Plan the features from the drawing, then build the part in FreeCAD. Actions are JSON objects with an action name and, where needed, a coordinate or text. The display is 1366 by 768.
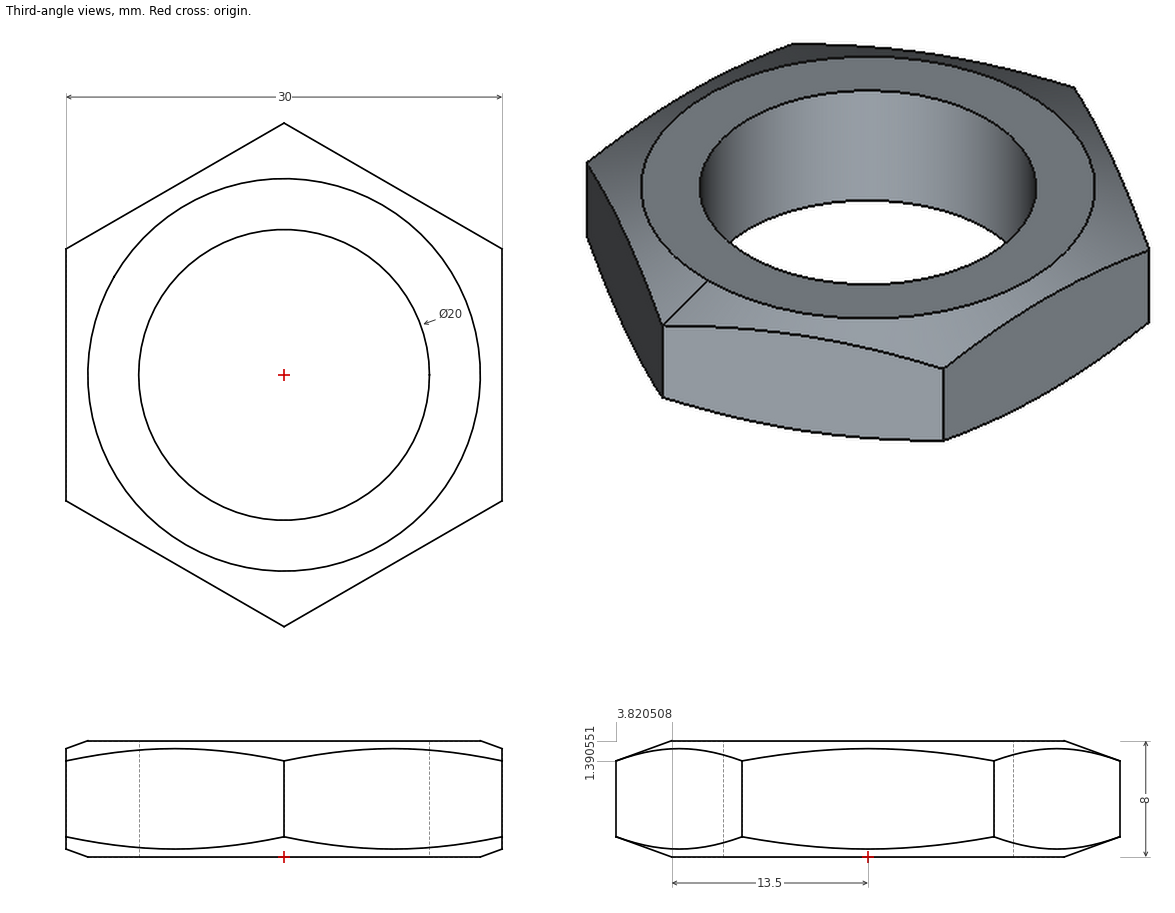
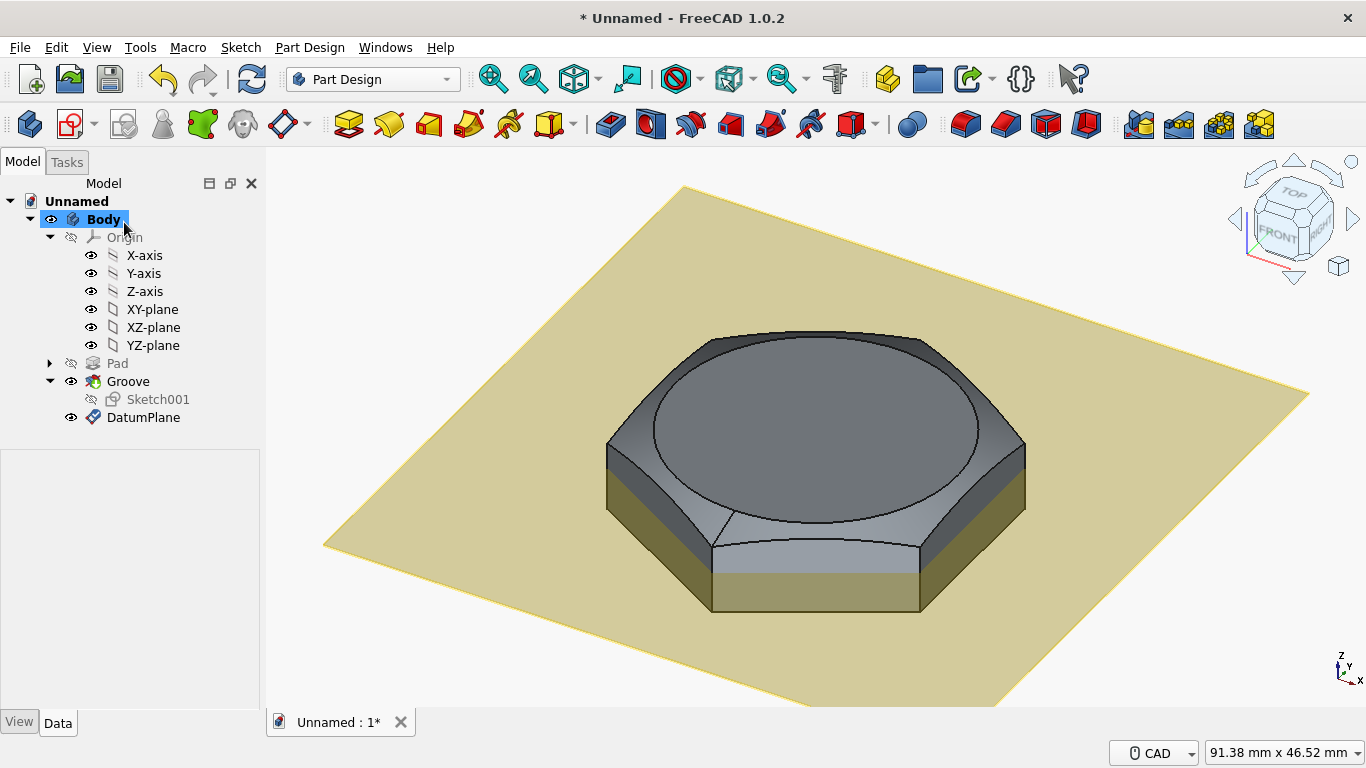
{"action": "left_click", "coordinate": [116, 381]}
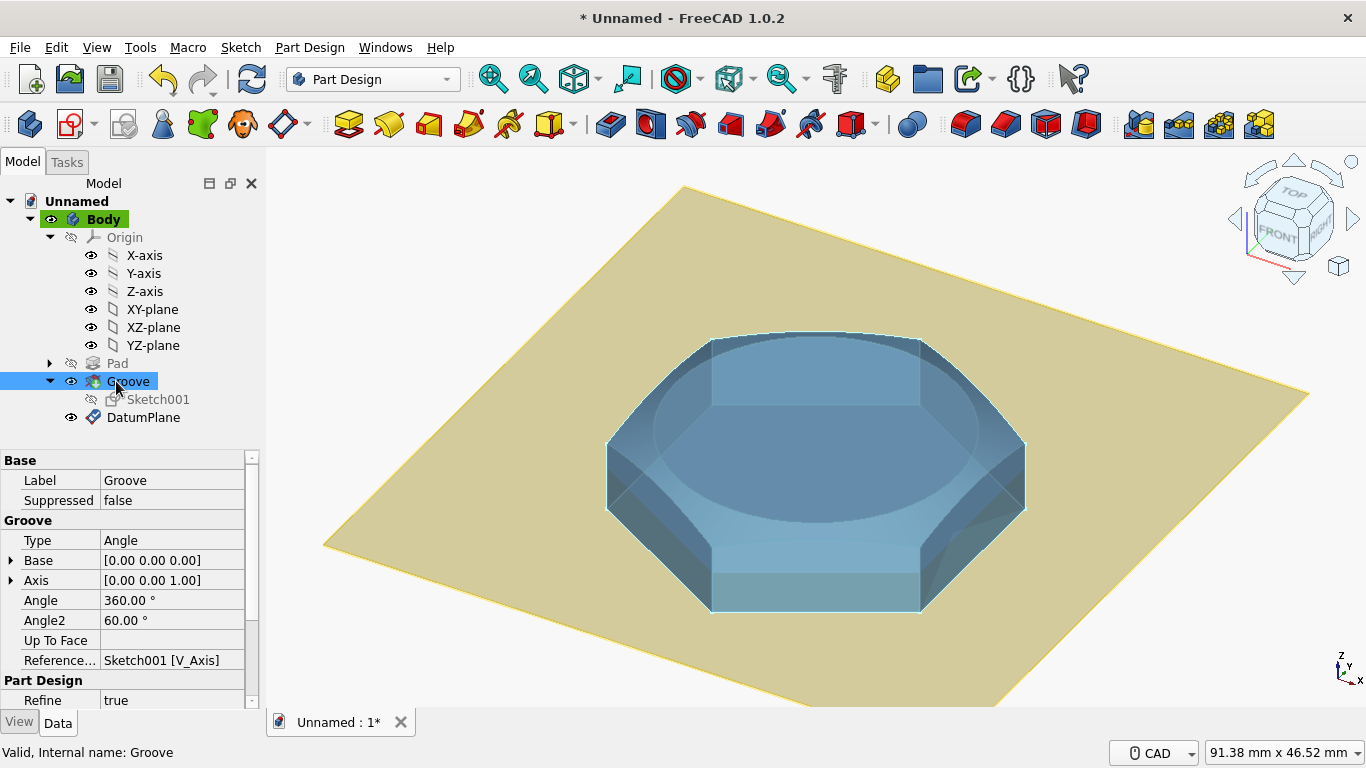
{"action": "left_click", "coordinate": [1140, 124]}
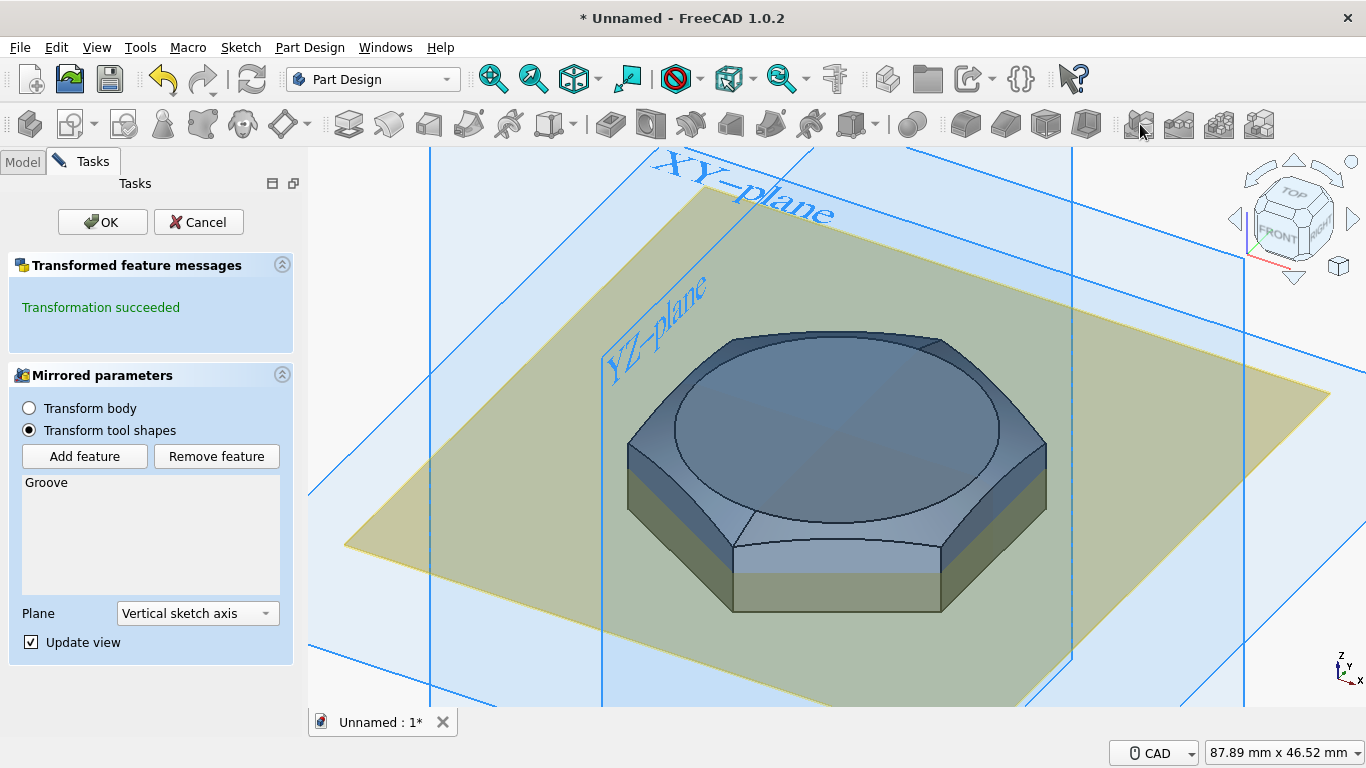
{"action": "left_click", "coordinate": [198, 614]}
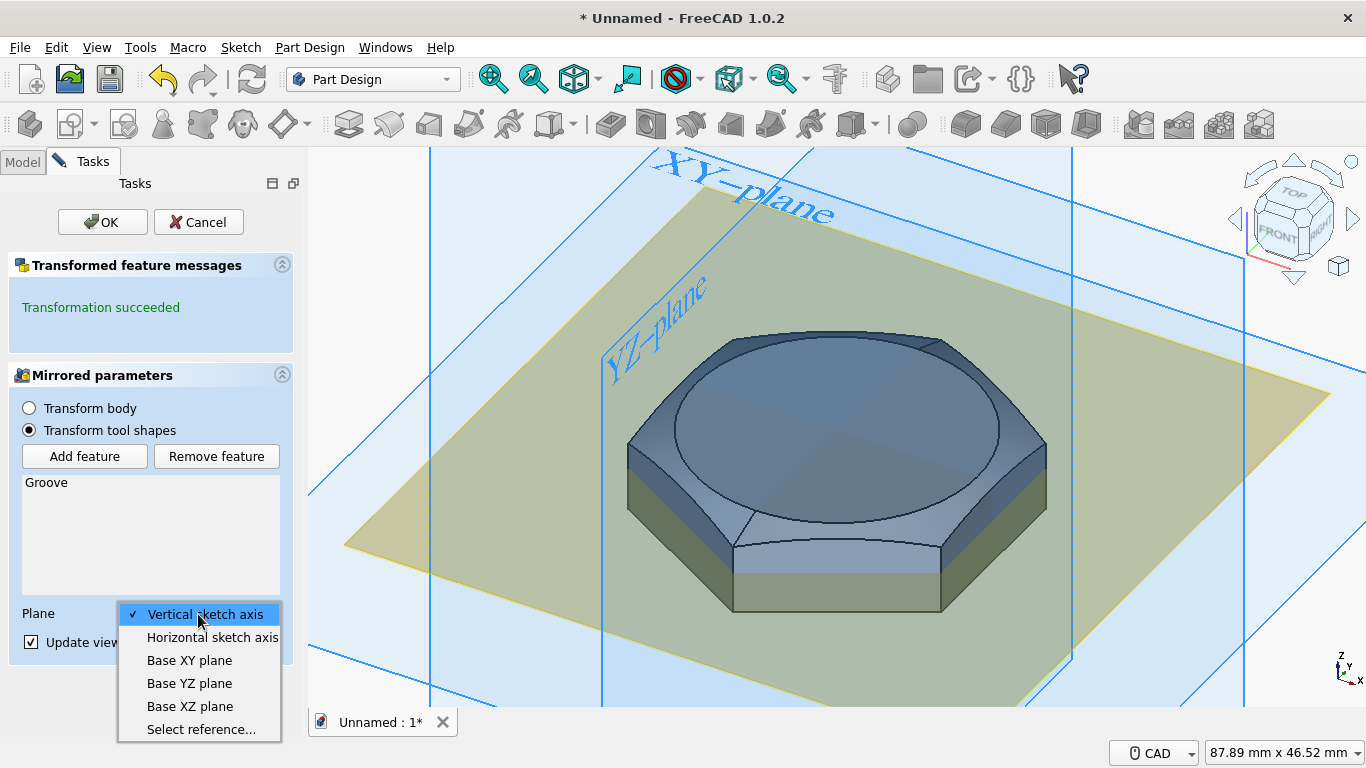
{"action": "left_click", "coordinate": [198, 730]}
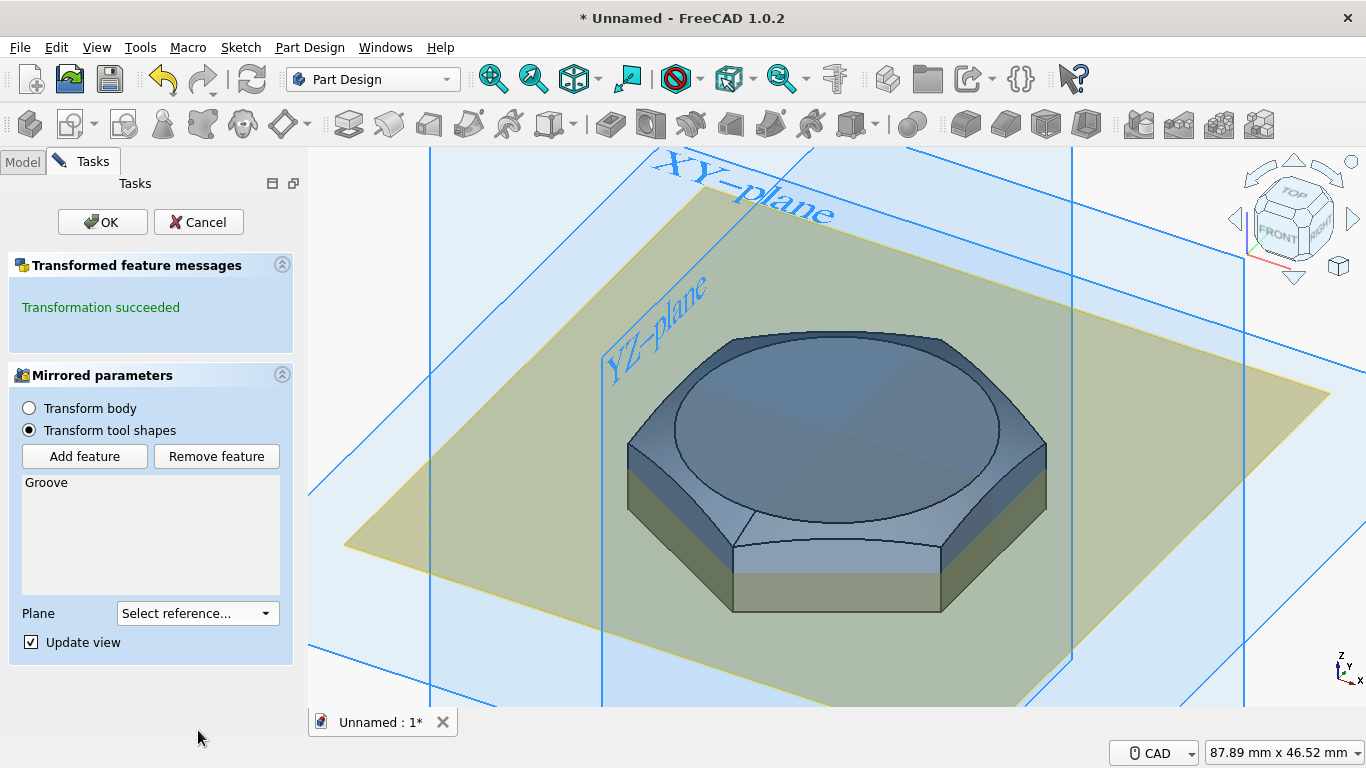
{"action": "left_click", "coordinate": [23, 161]}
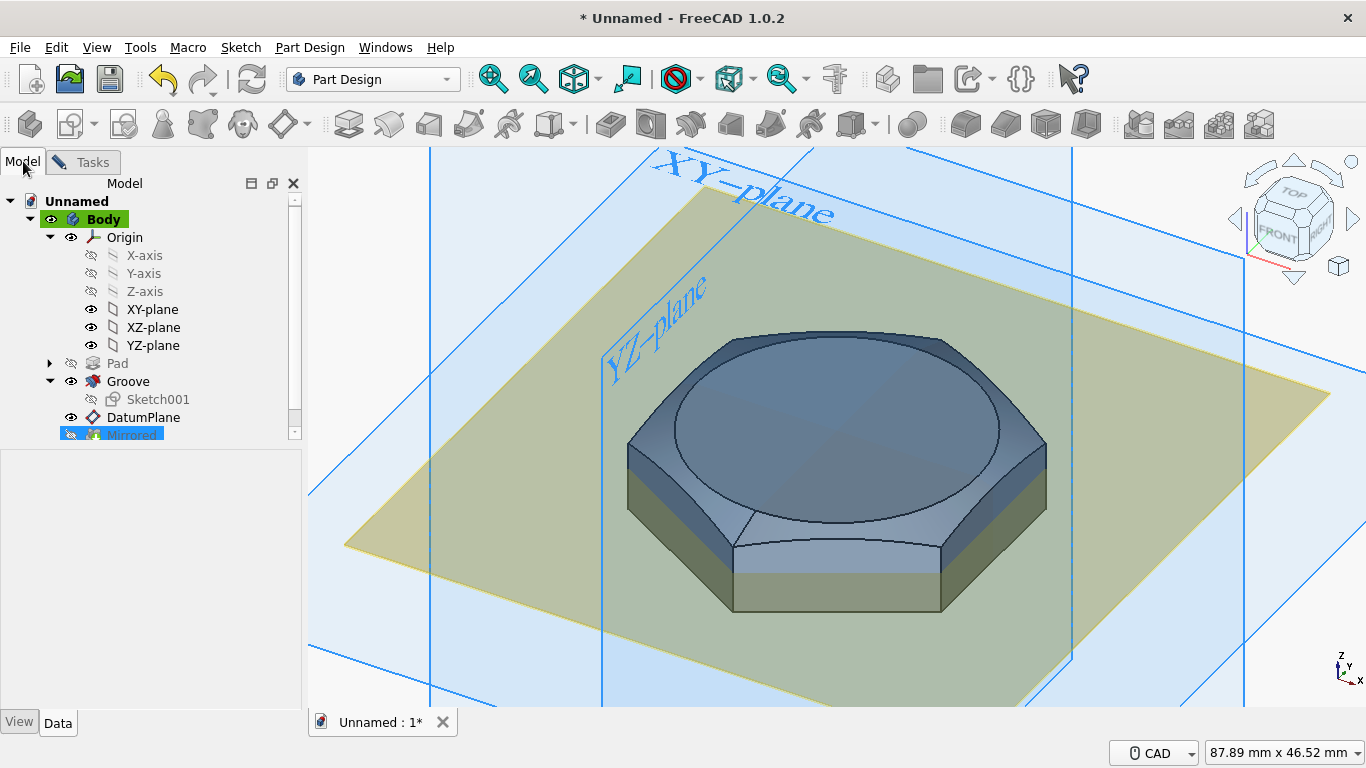
{"action": "left_click", "coordinate": [116, 417]}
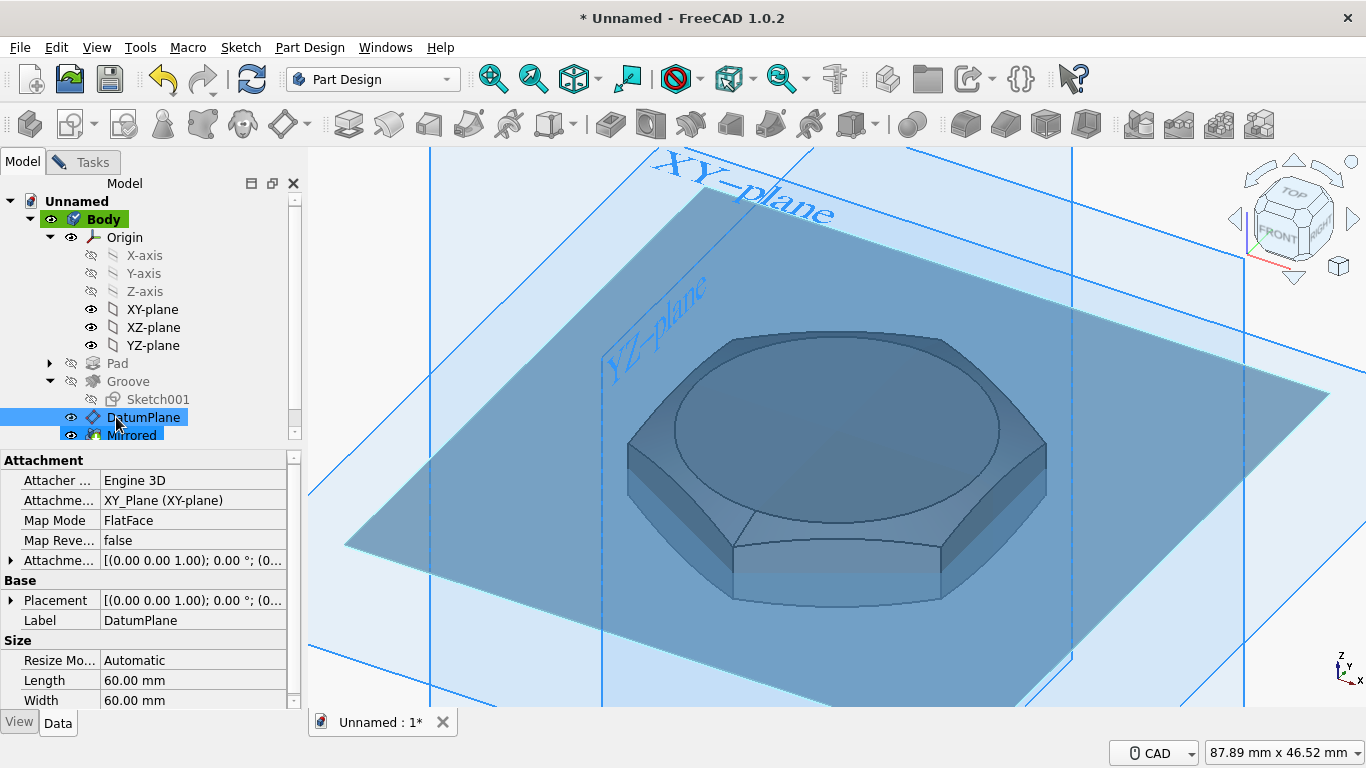
{"action": "left_click", "coordinate": [84, 161]}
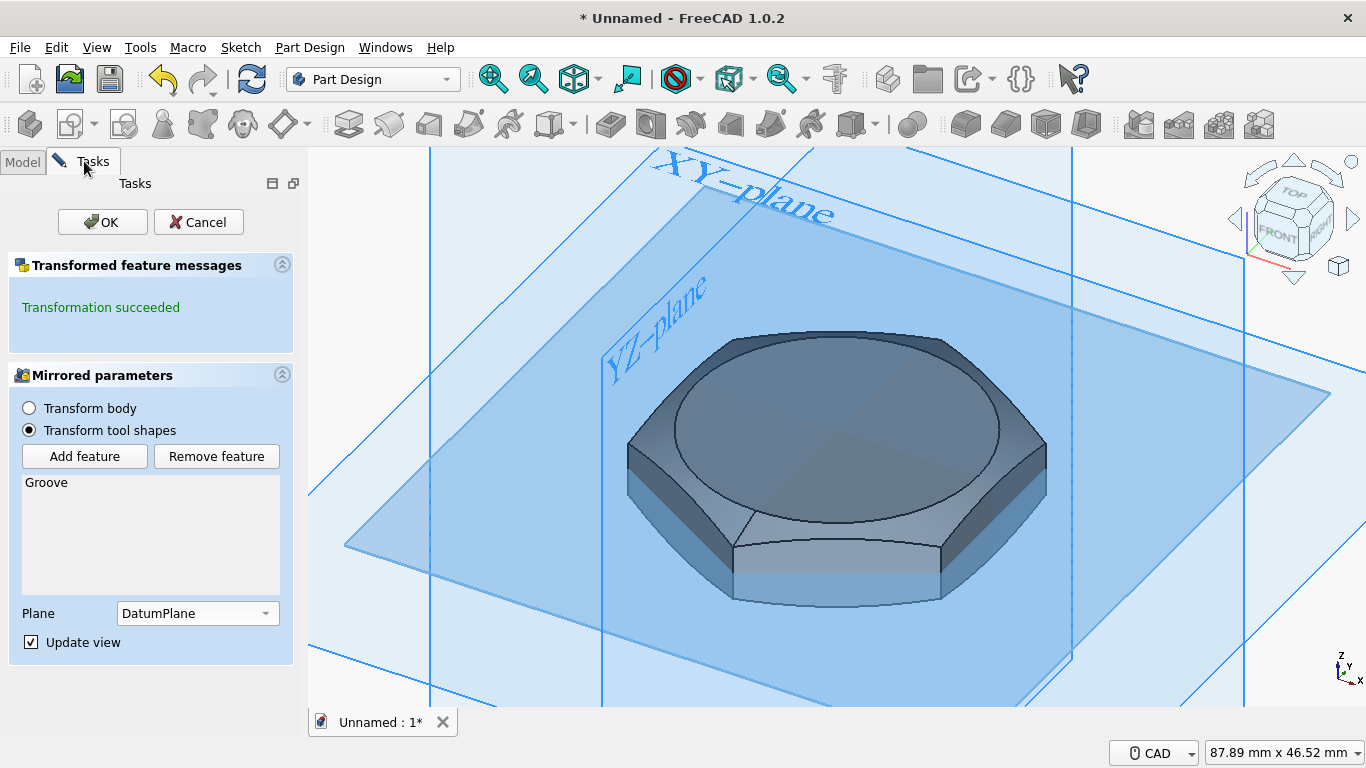
{"action": "left_click", "coordinate": [103, 222]}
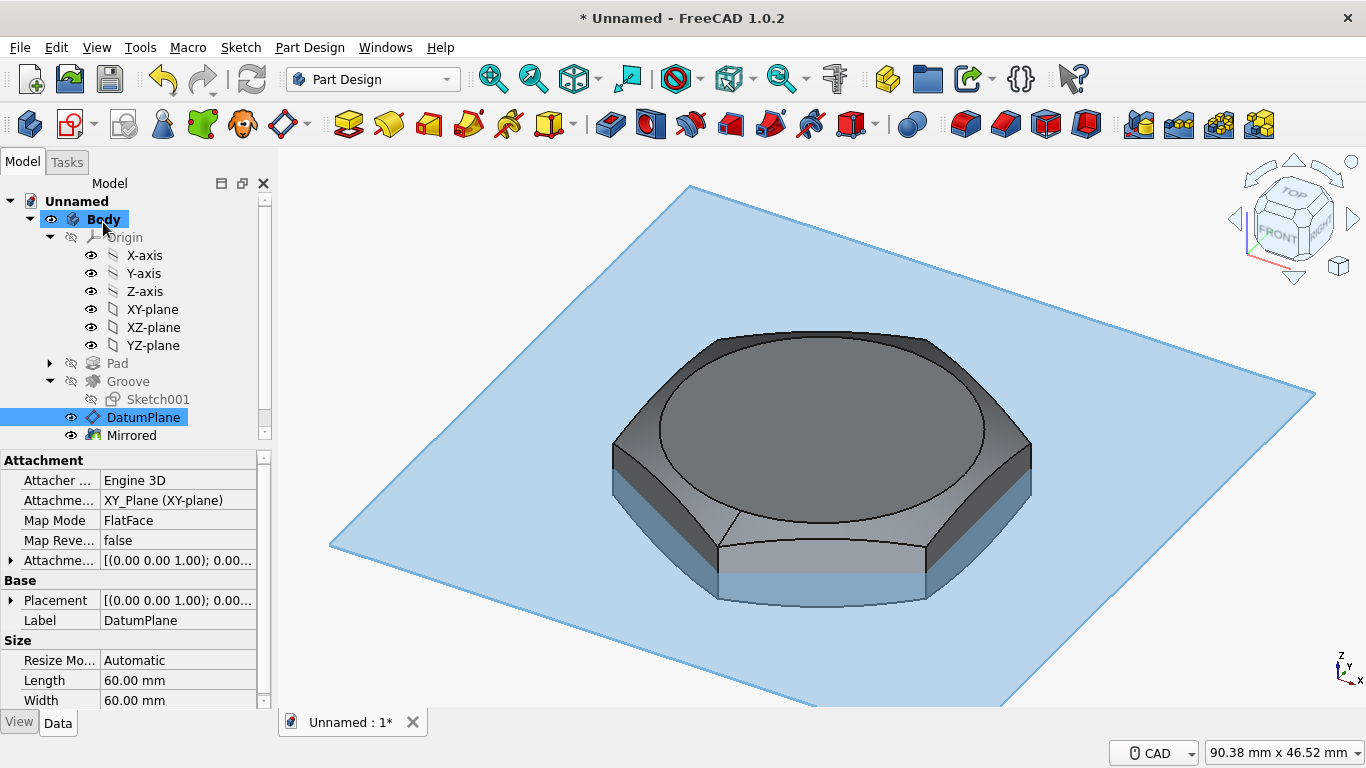
{"action": "left_click", "coordinate": [116, 417]}
{"action": "key", "text": "space"}